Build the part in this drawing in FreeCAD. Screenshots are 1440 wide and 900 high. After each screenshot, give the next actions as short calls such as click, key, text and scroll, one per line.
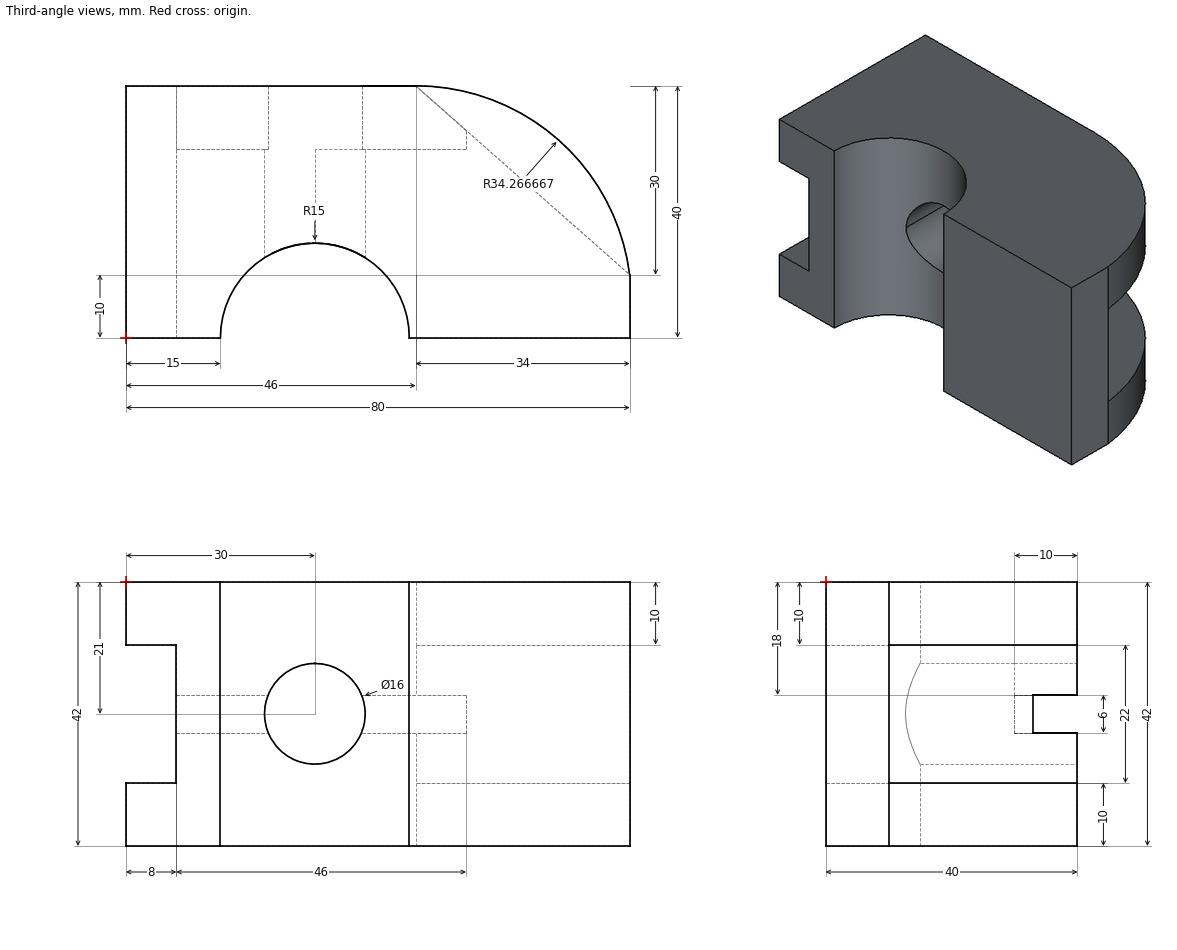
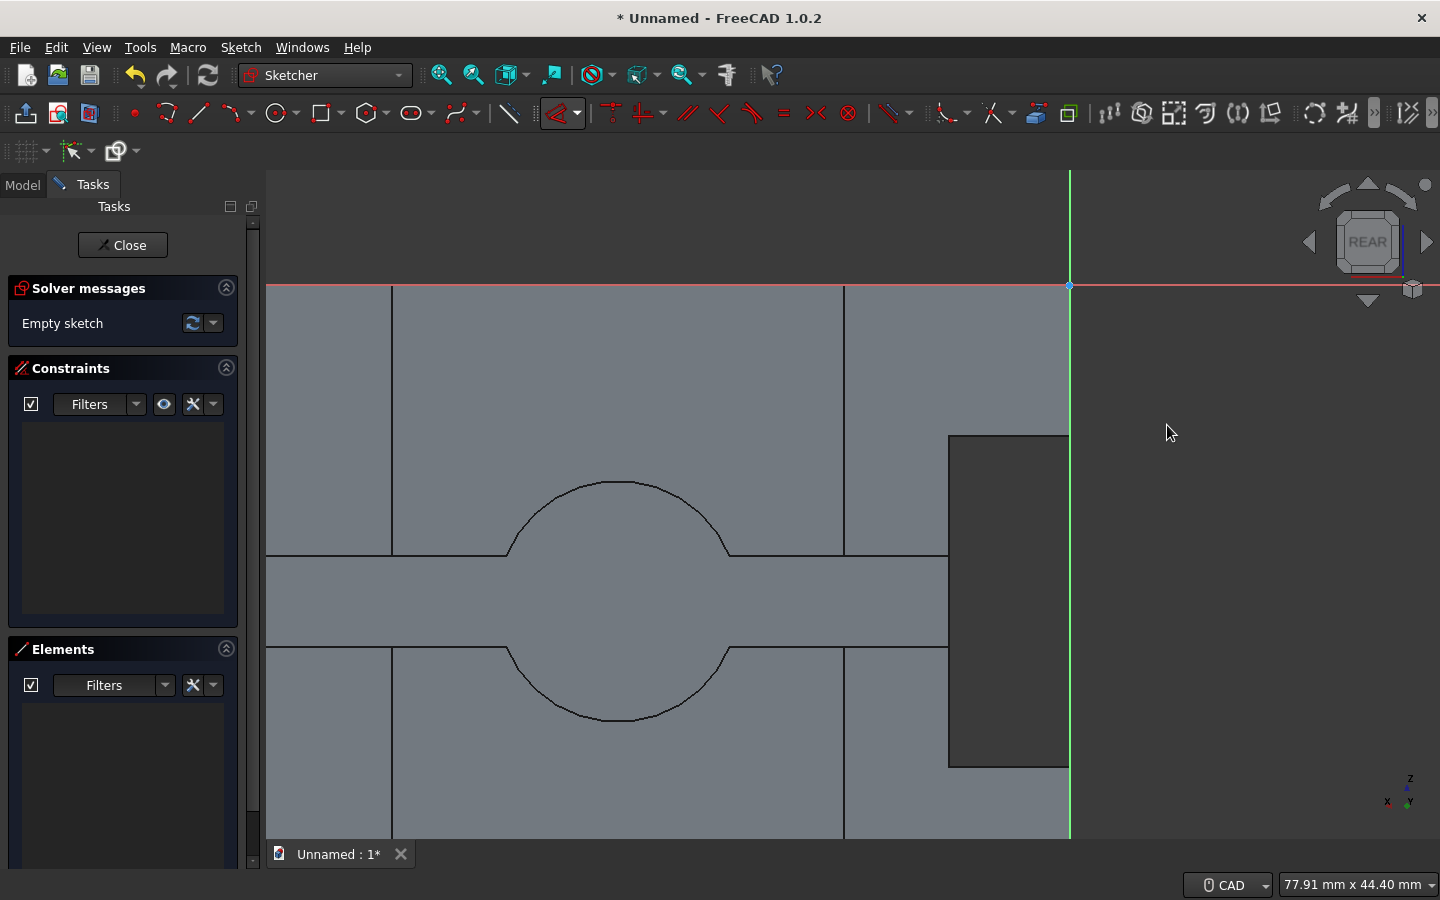
click(276, 114)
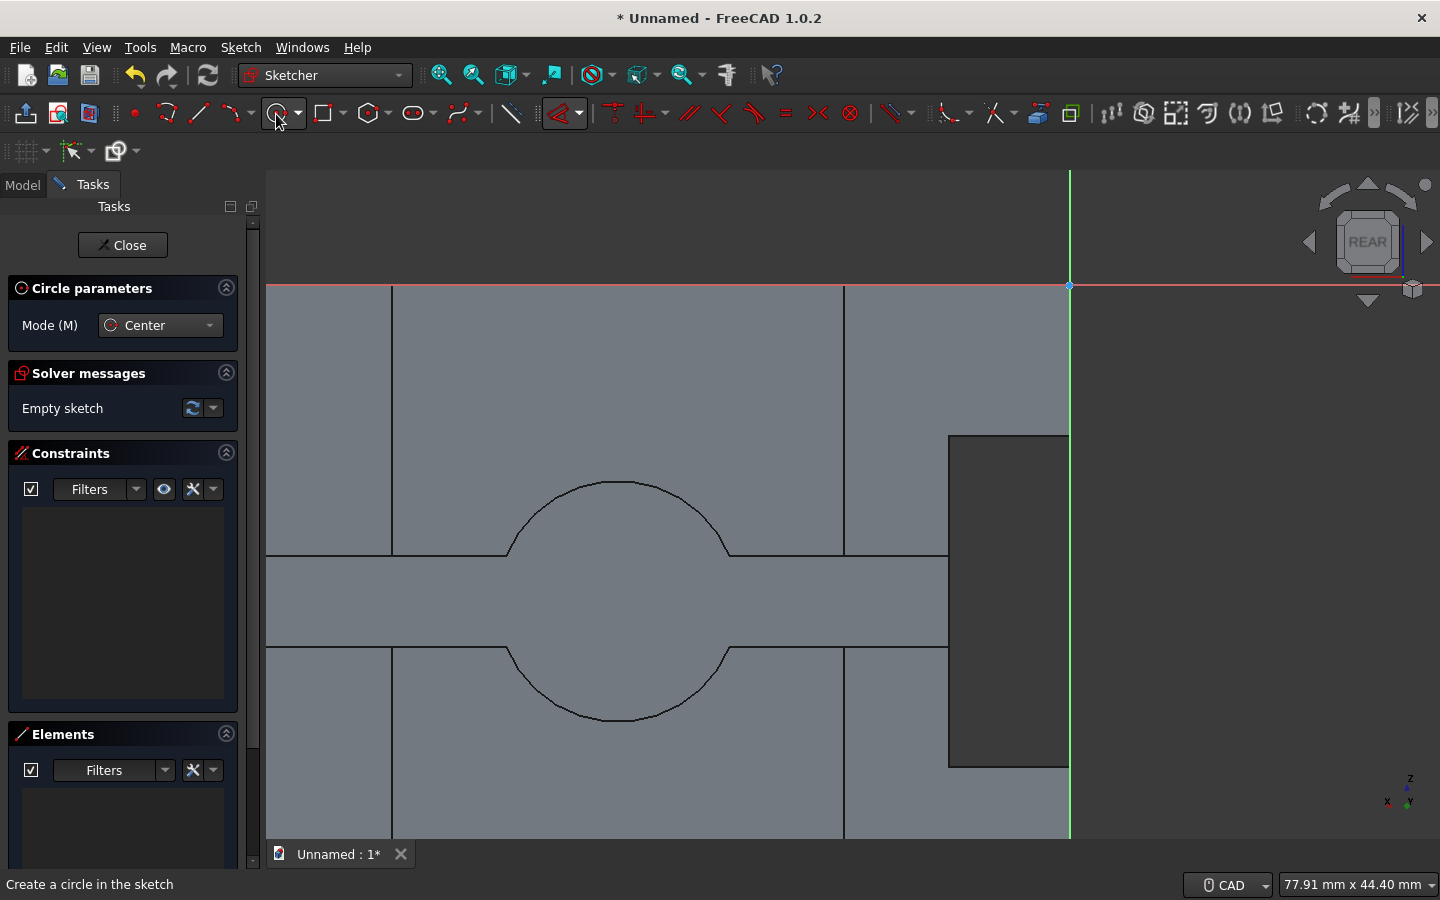
click(618, 601)
move(703, 516)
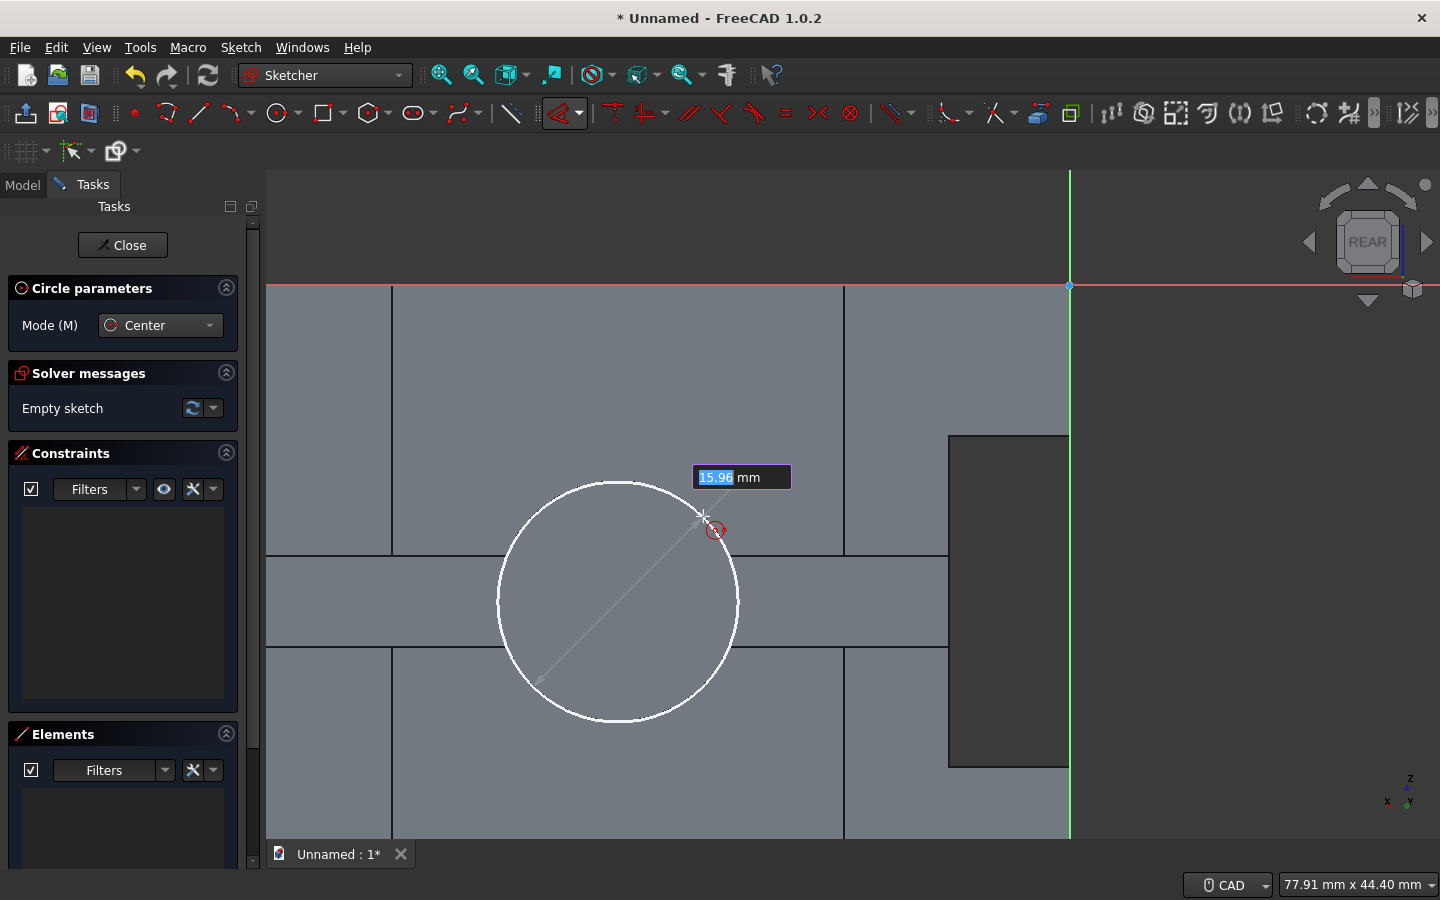
text(16)
key(Return)
key(Escape)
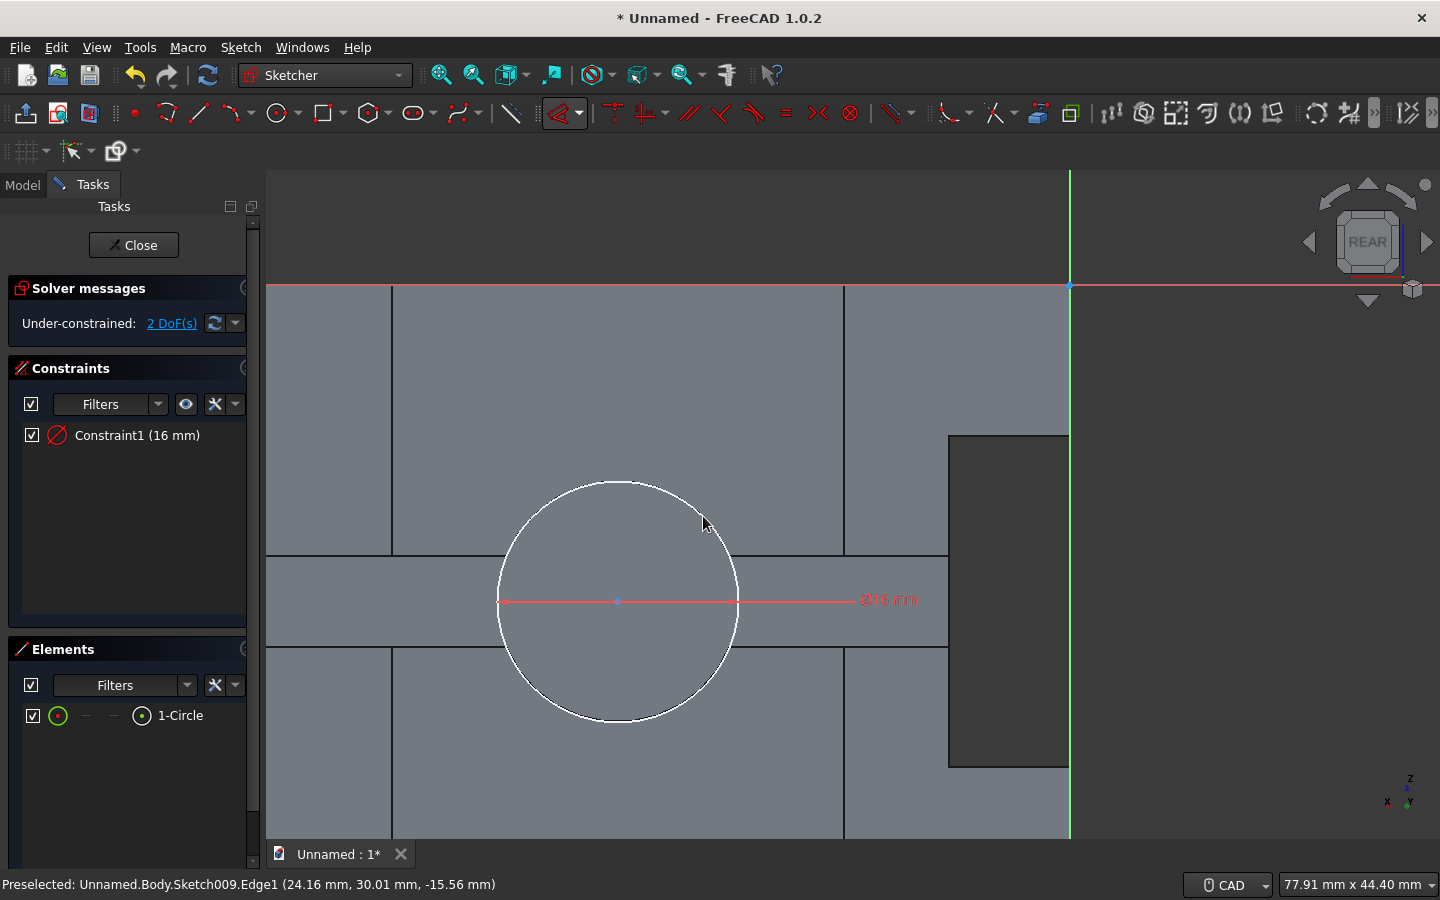
click(618, 602)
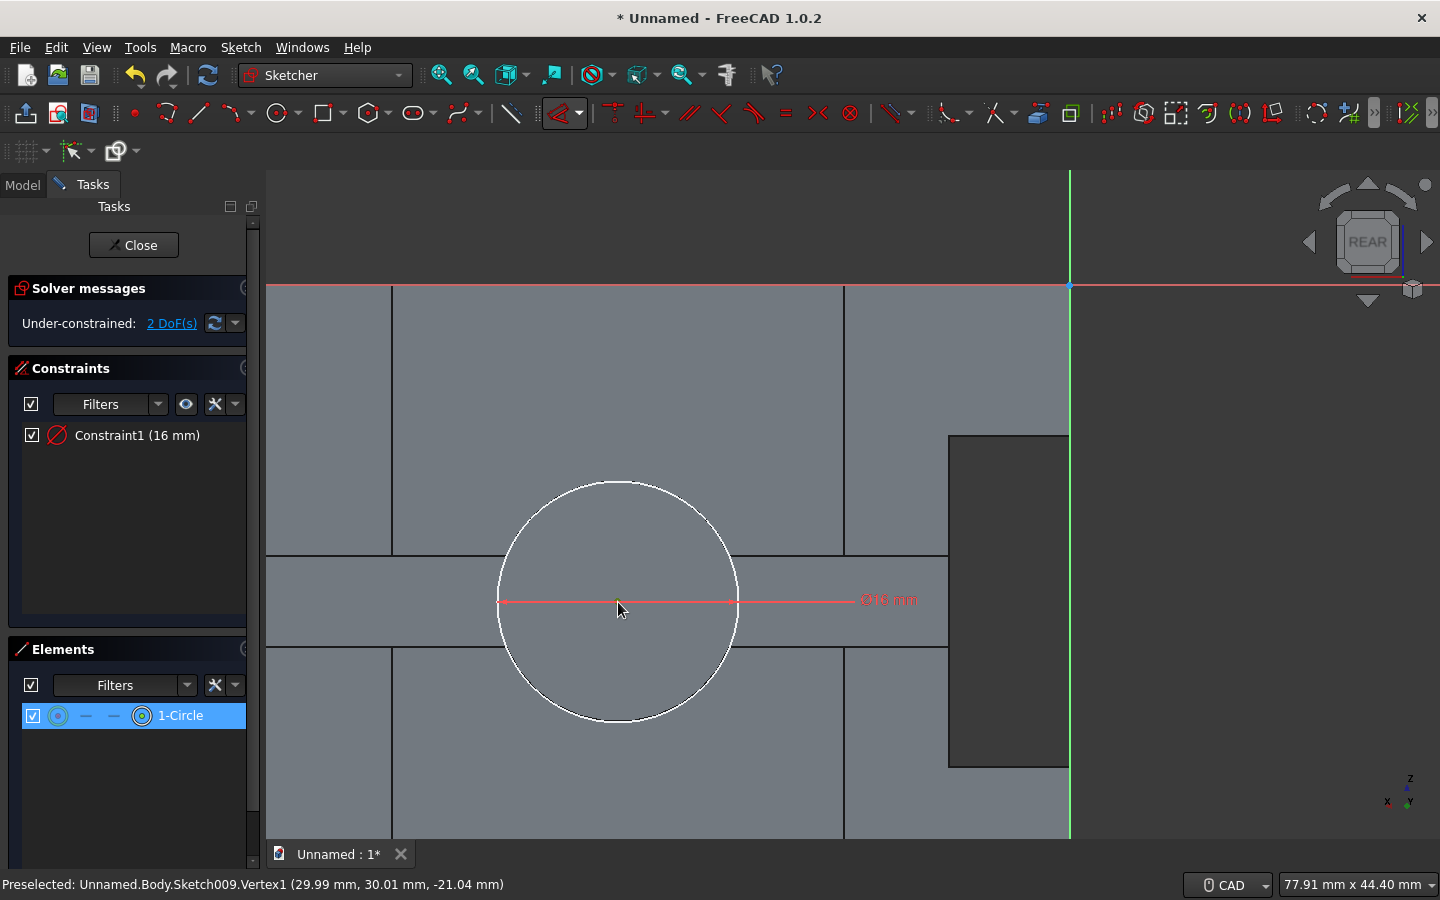
key(l)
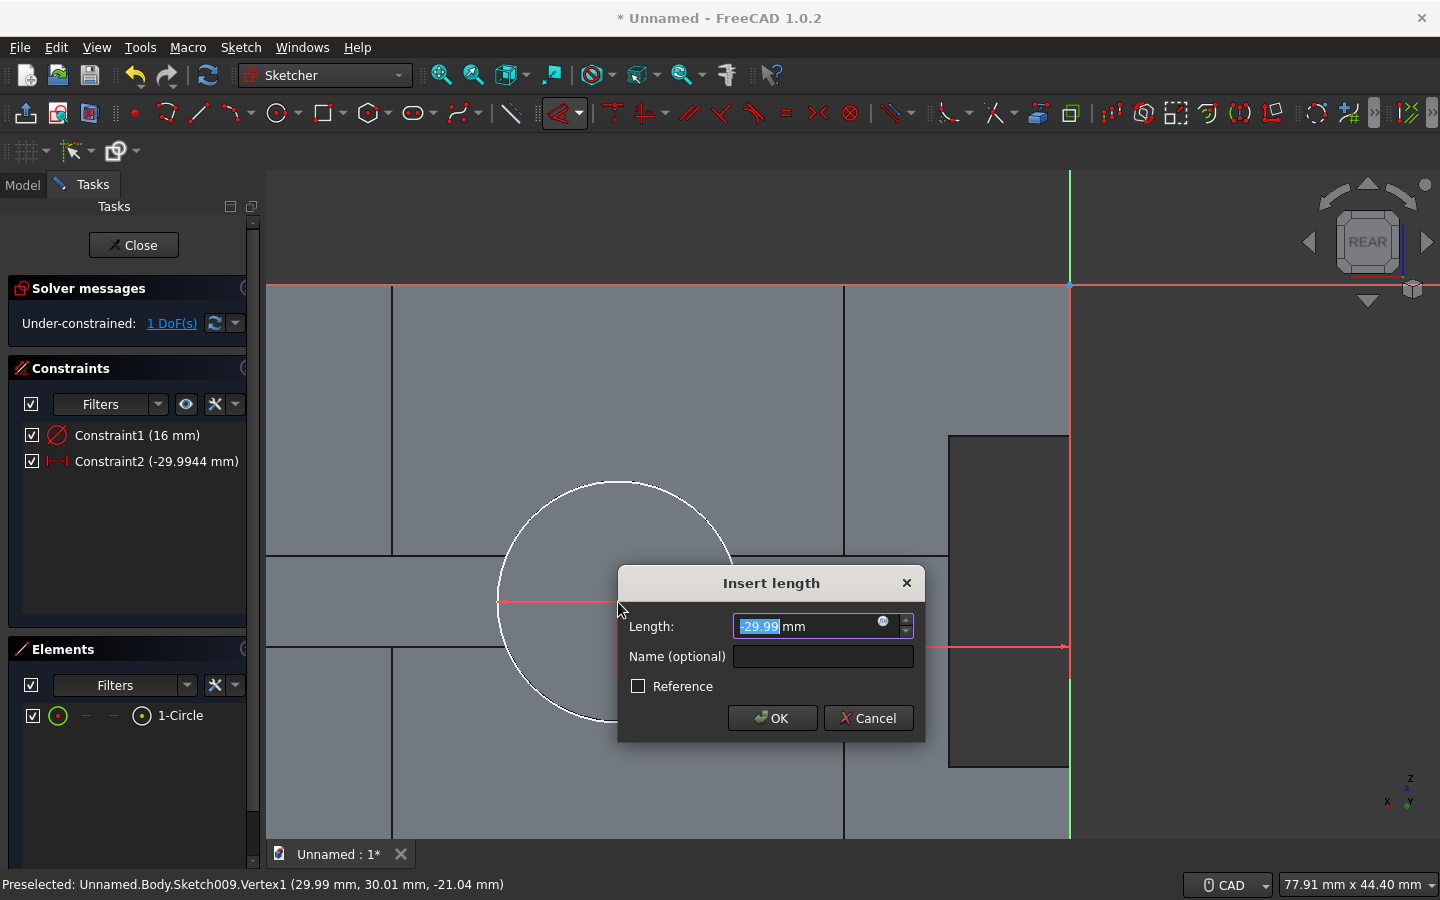
text(-30)
key(Return)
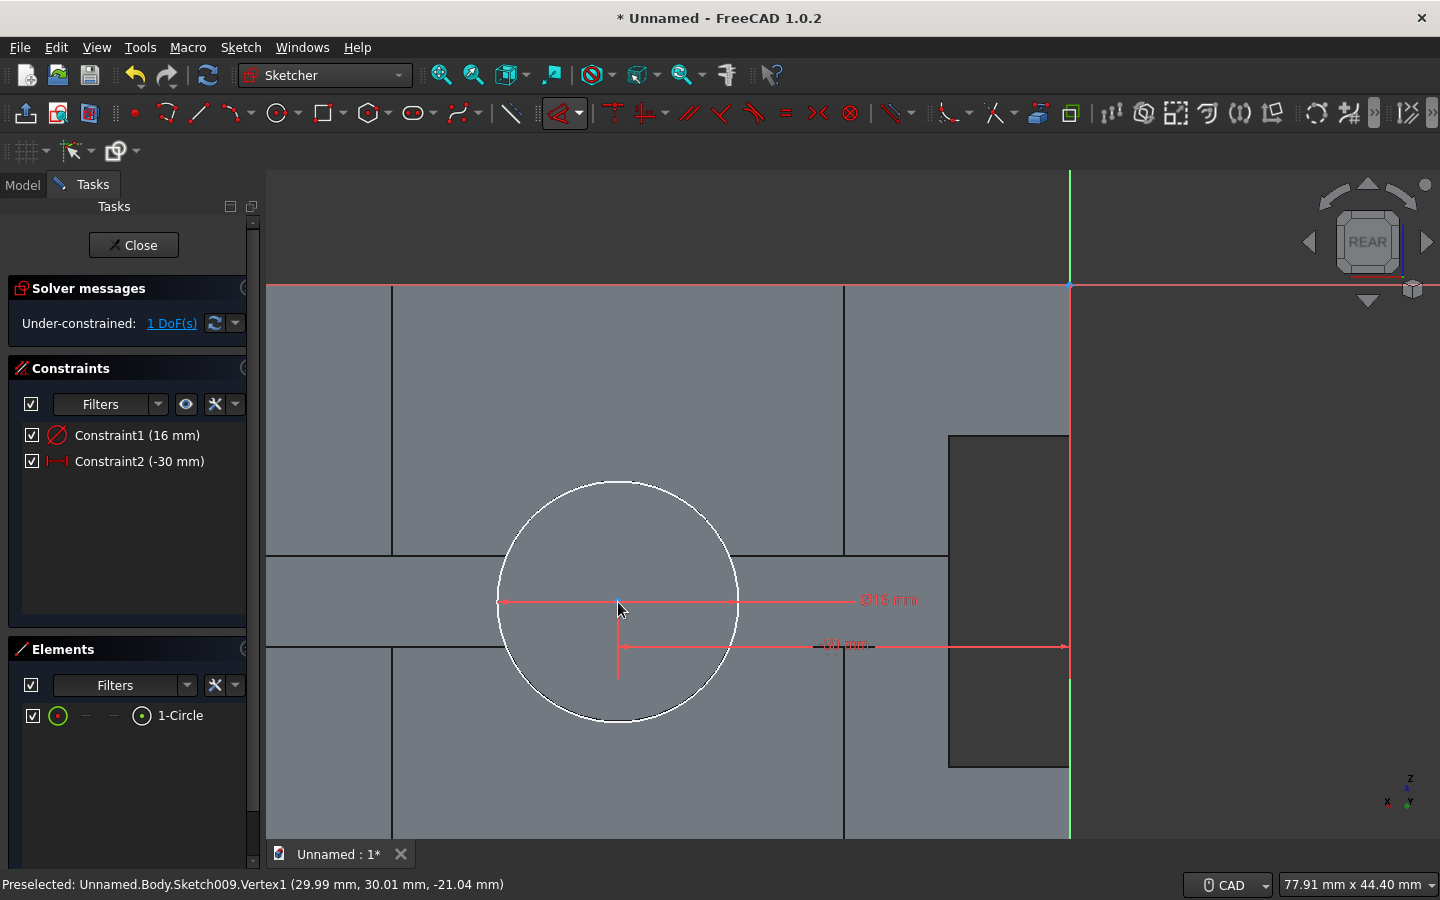
click(618, 602)